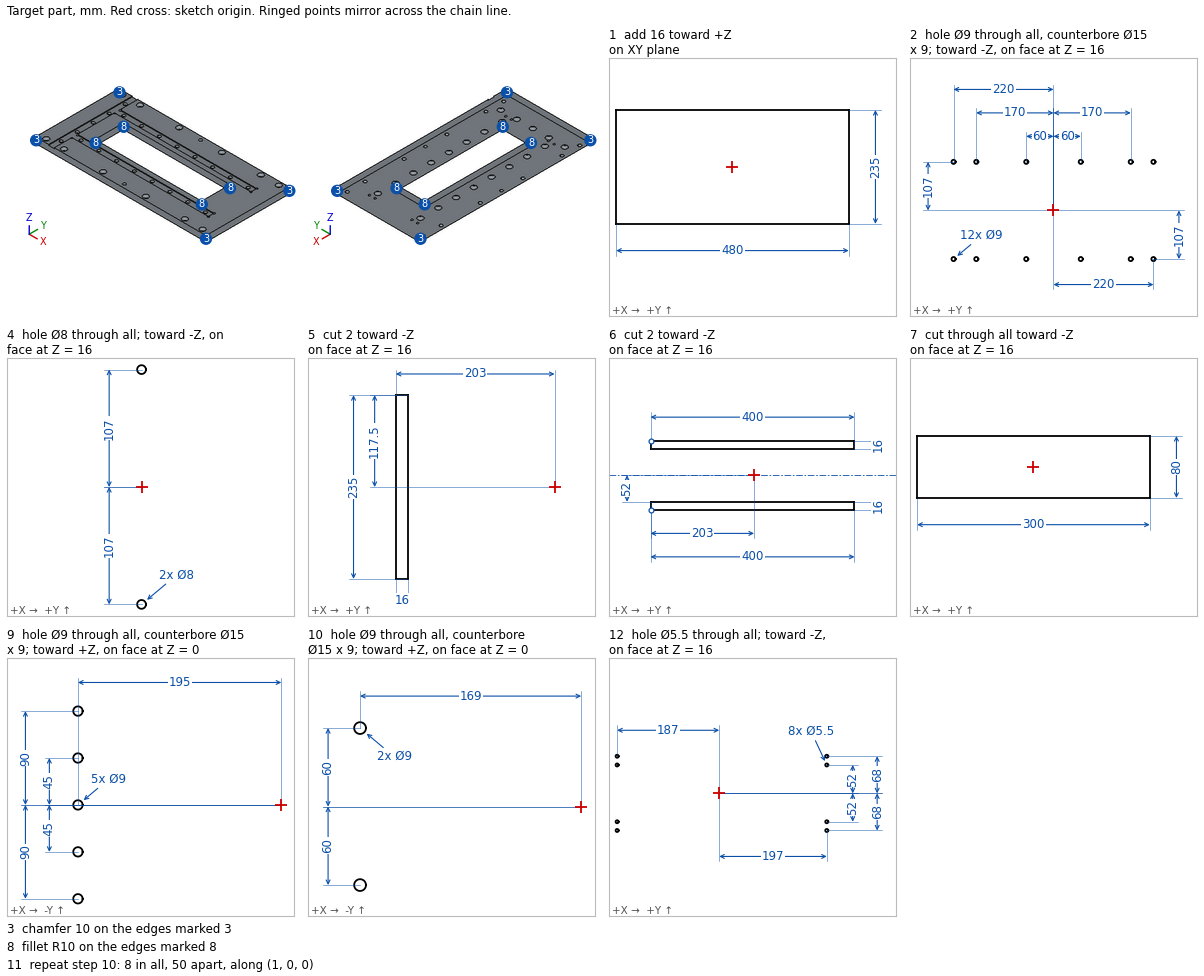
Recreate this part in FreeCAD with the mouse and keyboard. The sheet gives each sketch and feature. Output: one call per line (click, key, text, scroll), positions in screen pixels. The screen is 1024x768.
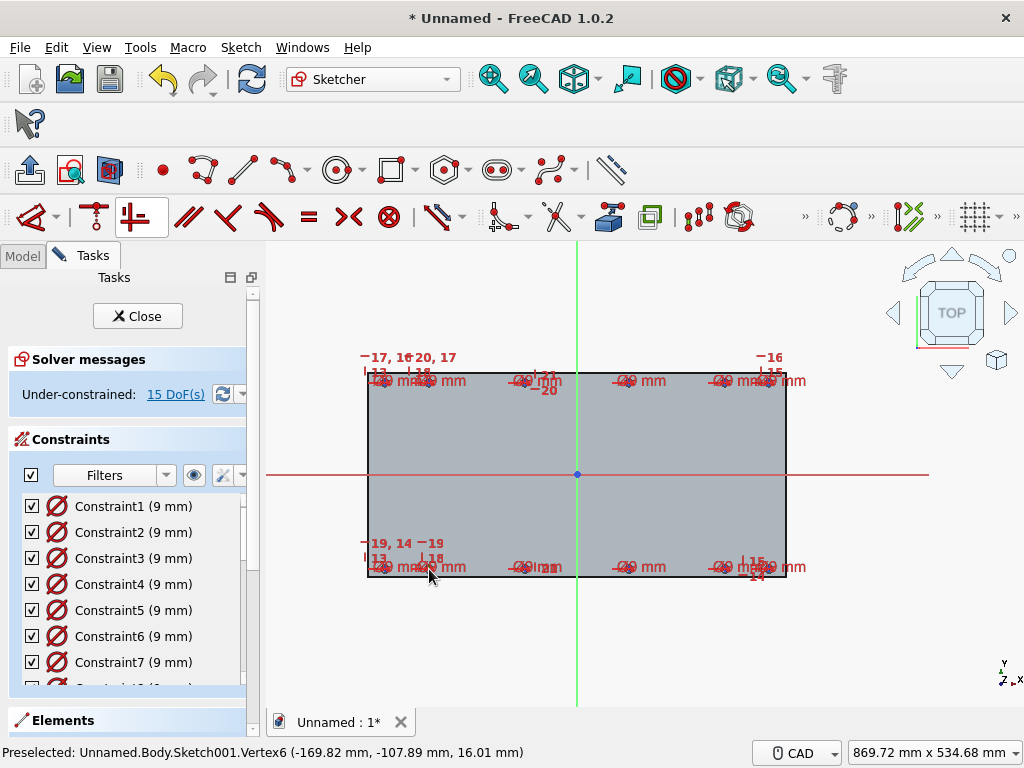
click(525, 569)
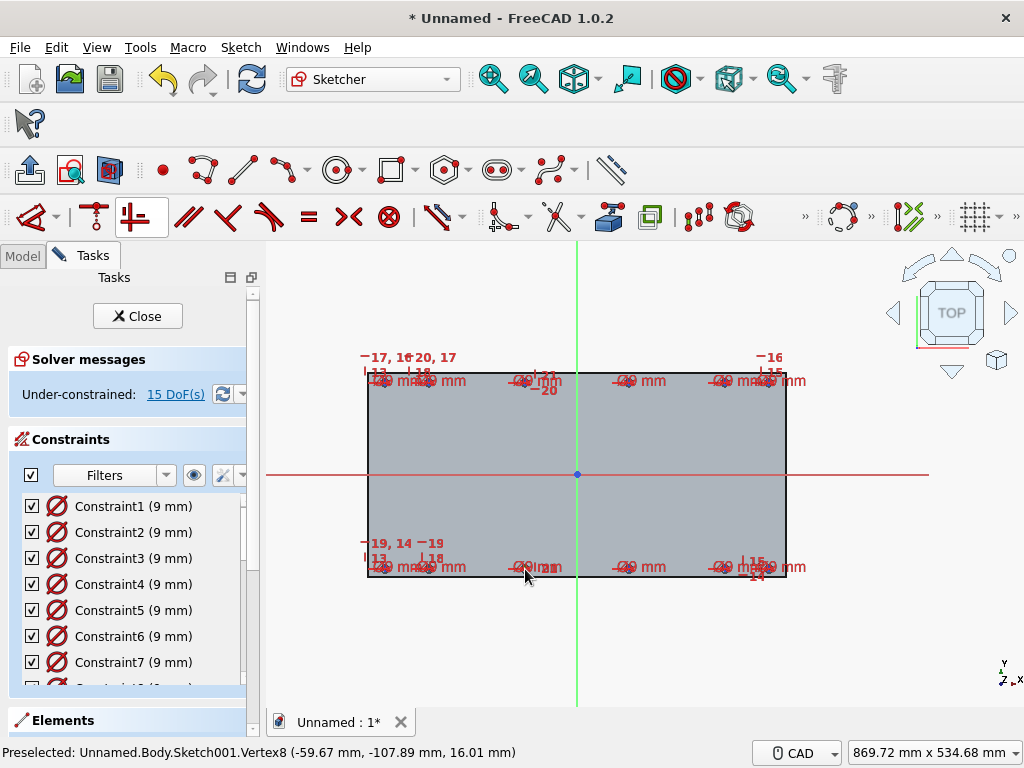
key(h)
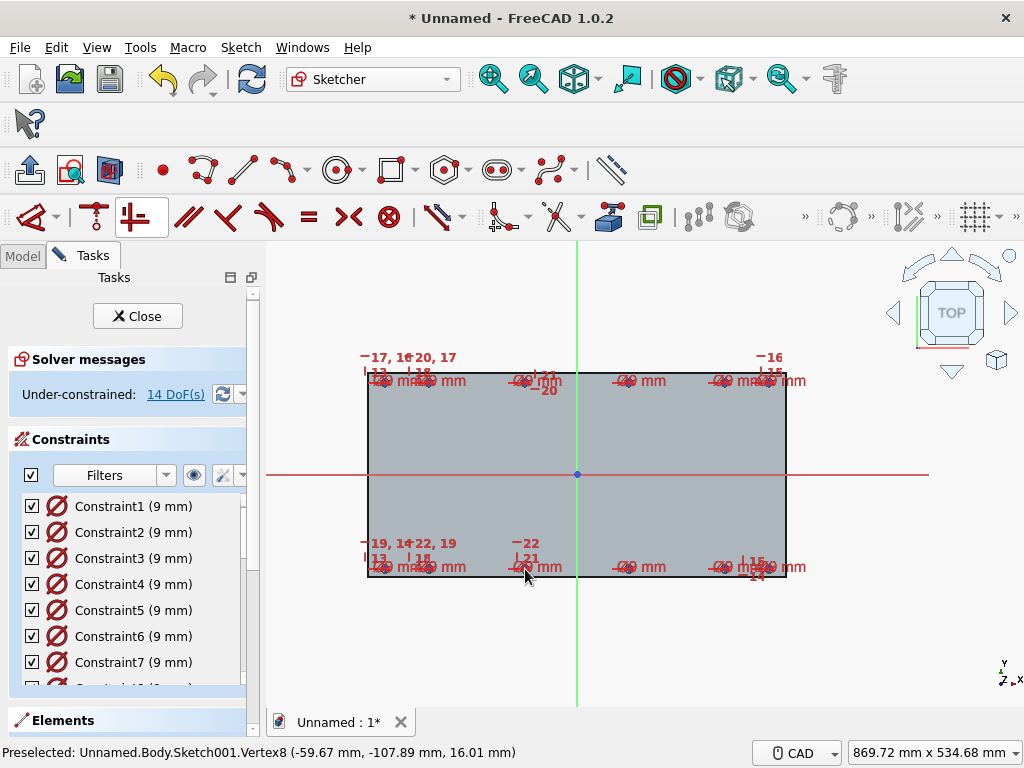
click(525, 383)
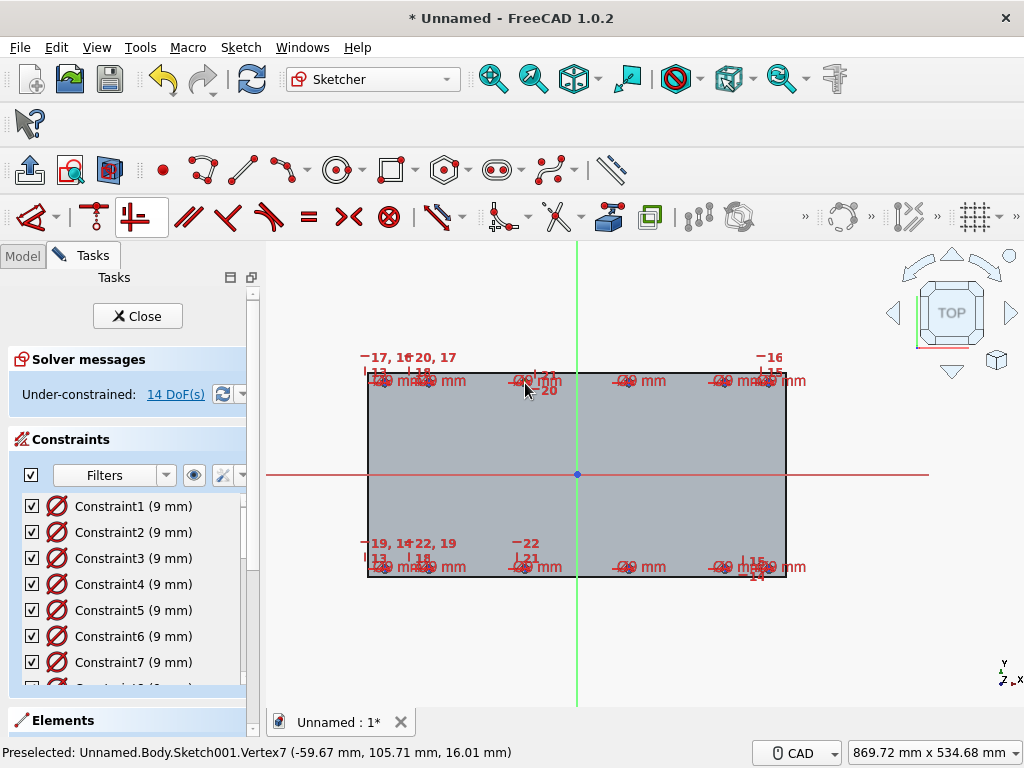
click(629, 383)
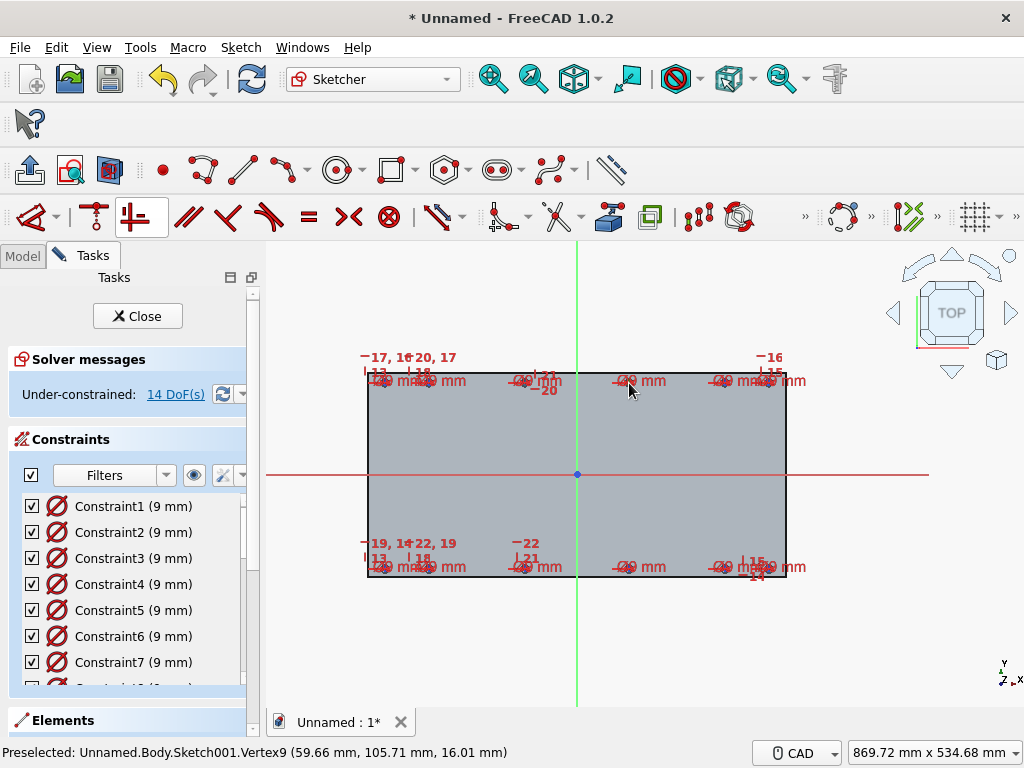
click(162, 218)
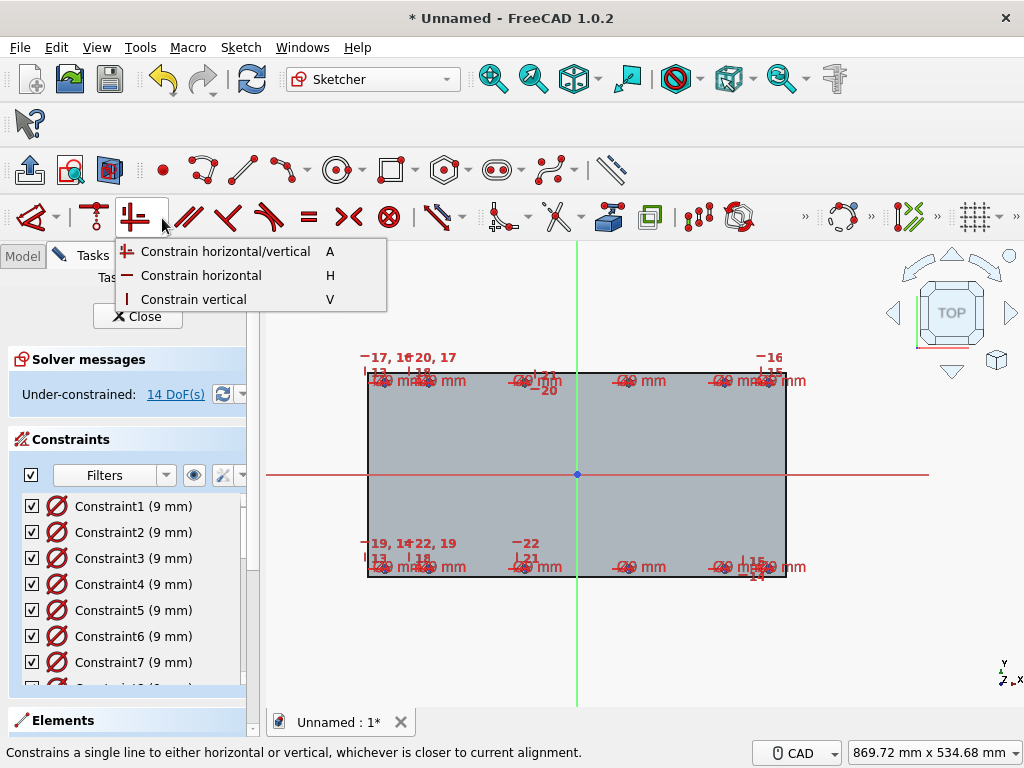
click(251, 275)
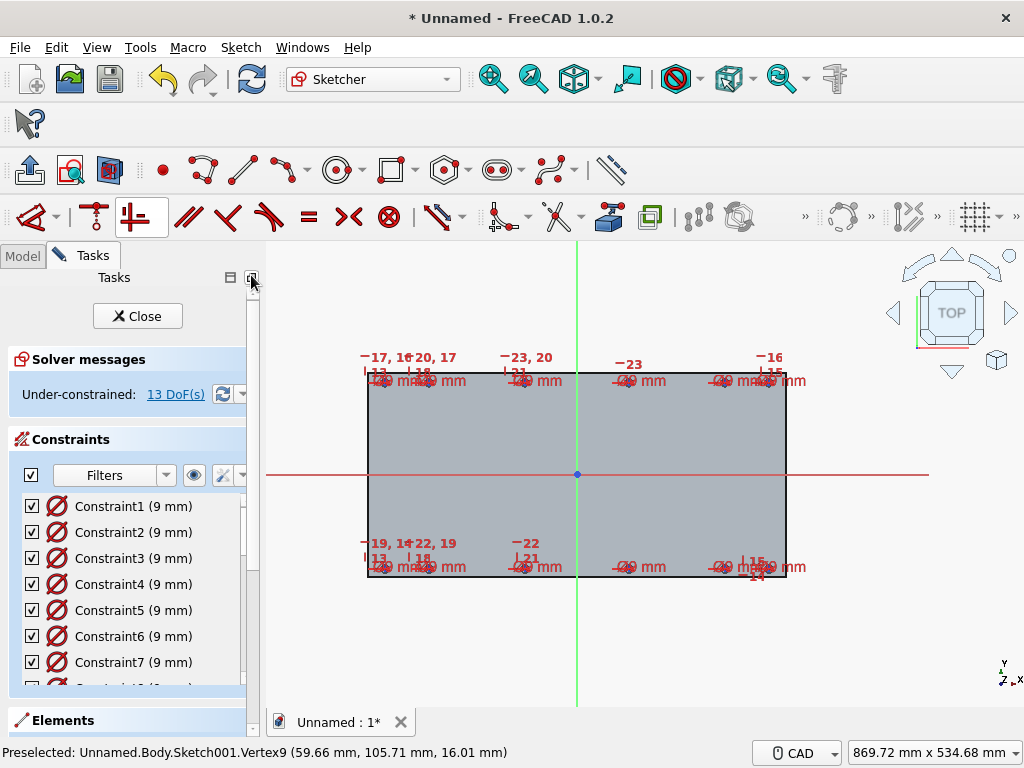
click(629, 383)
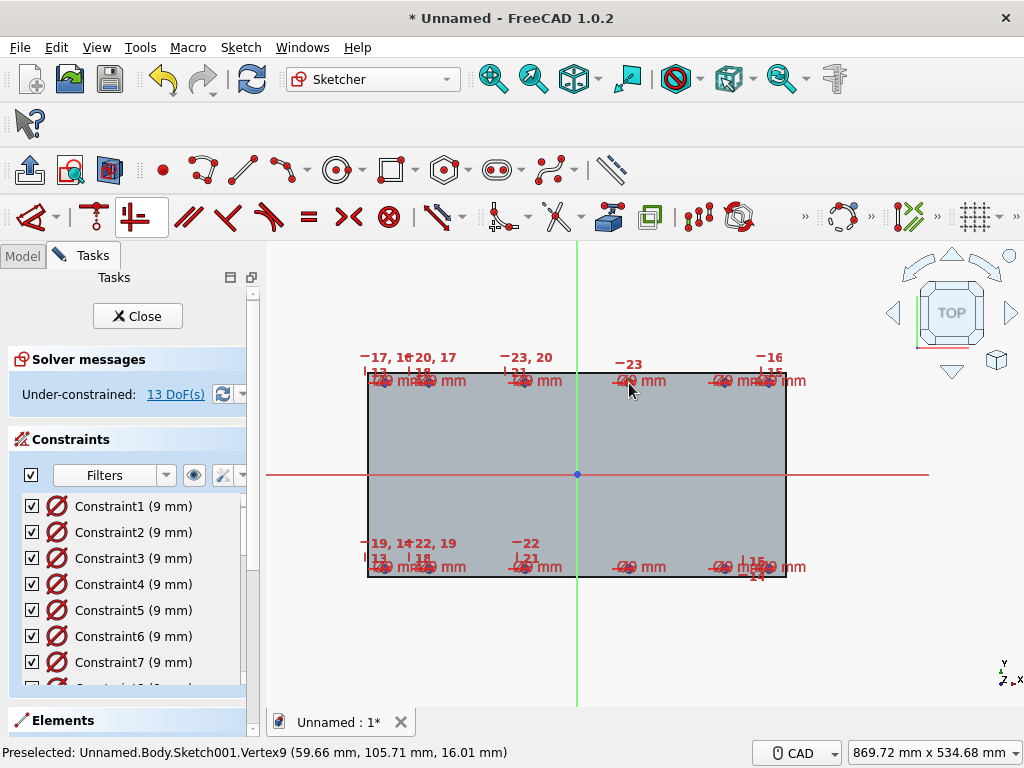
click(629, 569)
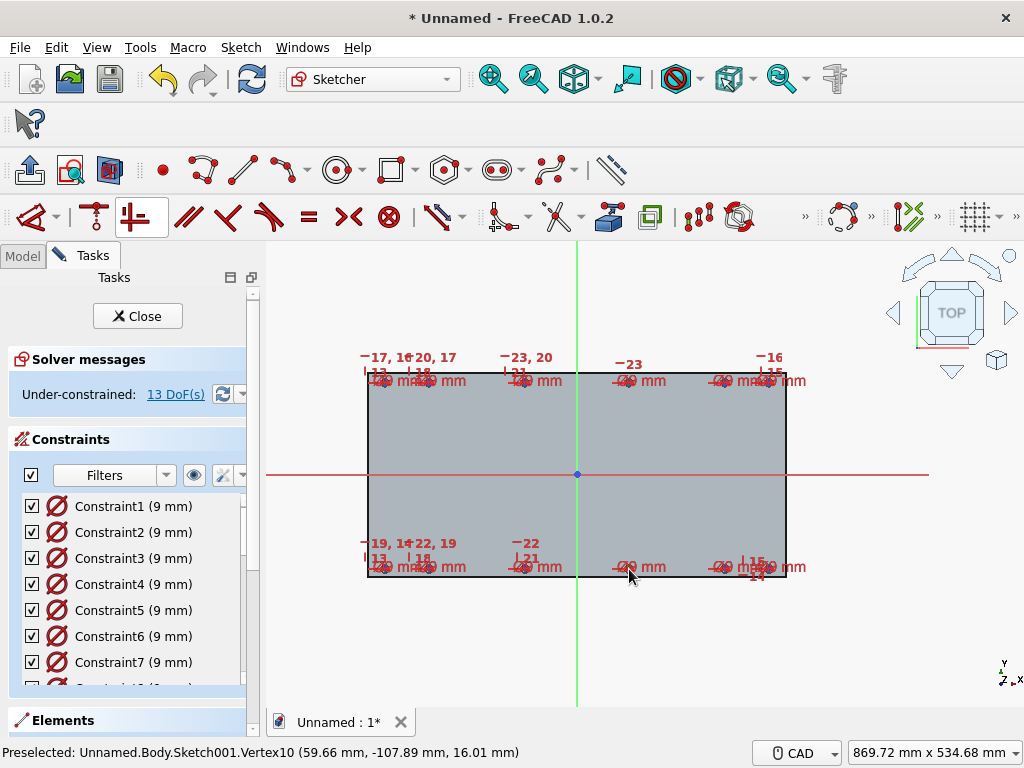
click(162, 218)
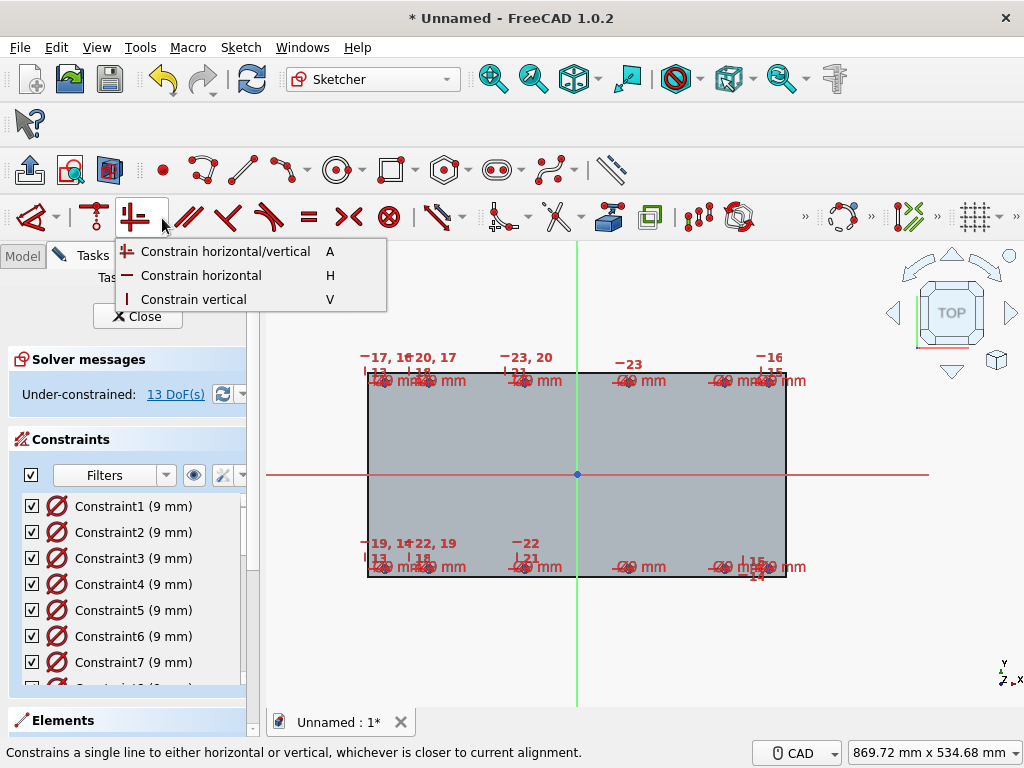
click(251, 299)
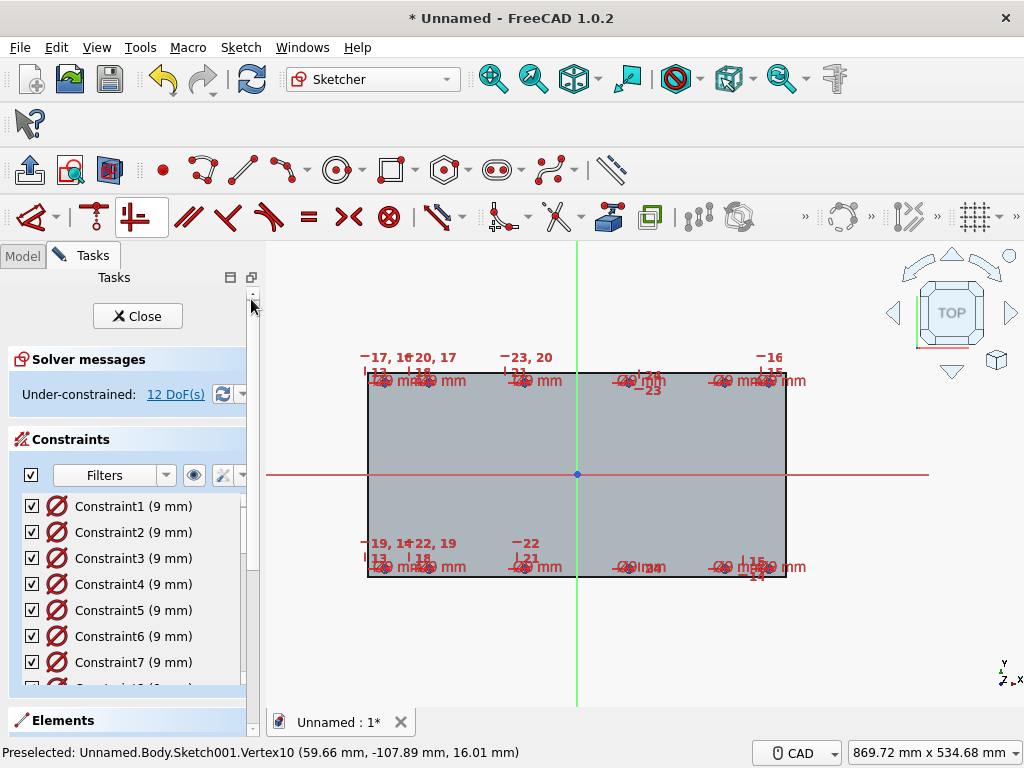
click(525, 569)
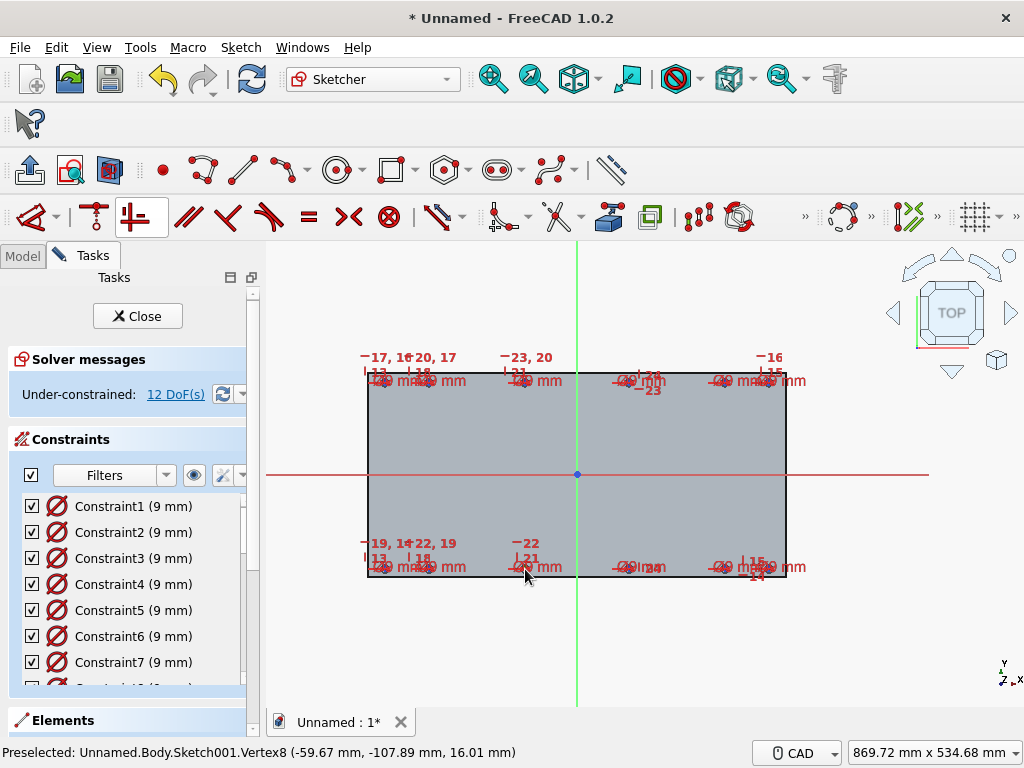
click(629, 569)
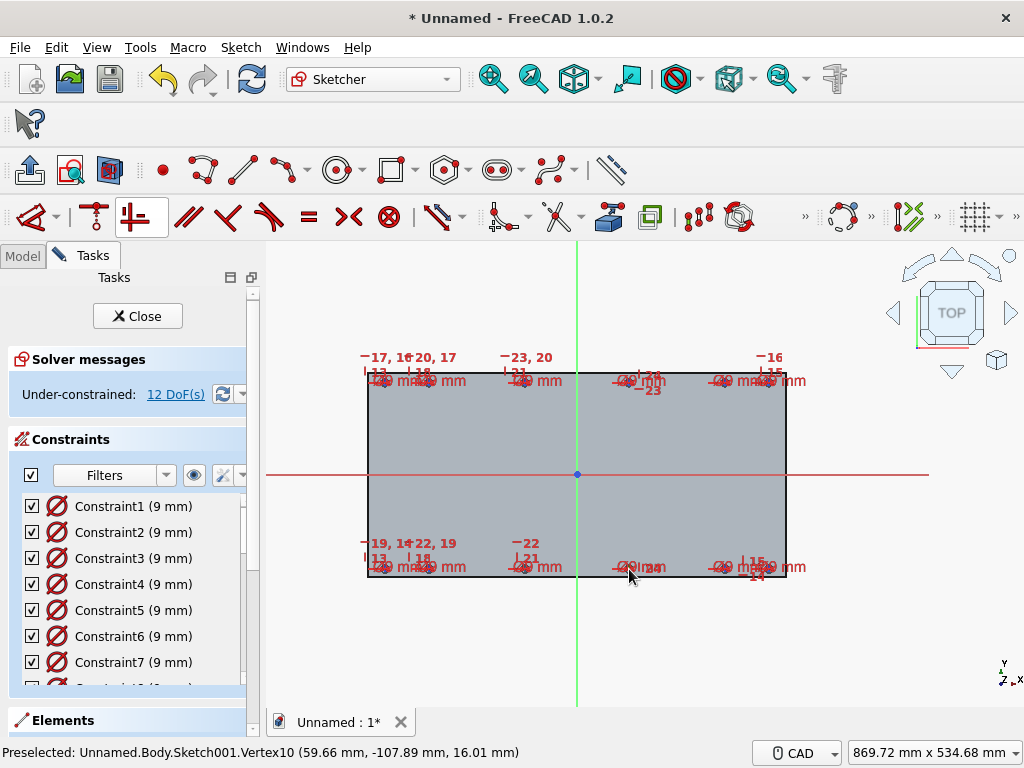
click(162, 218)